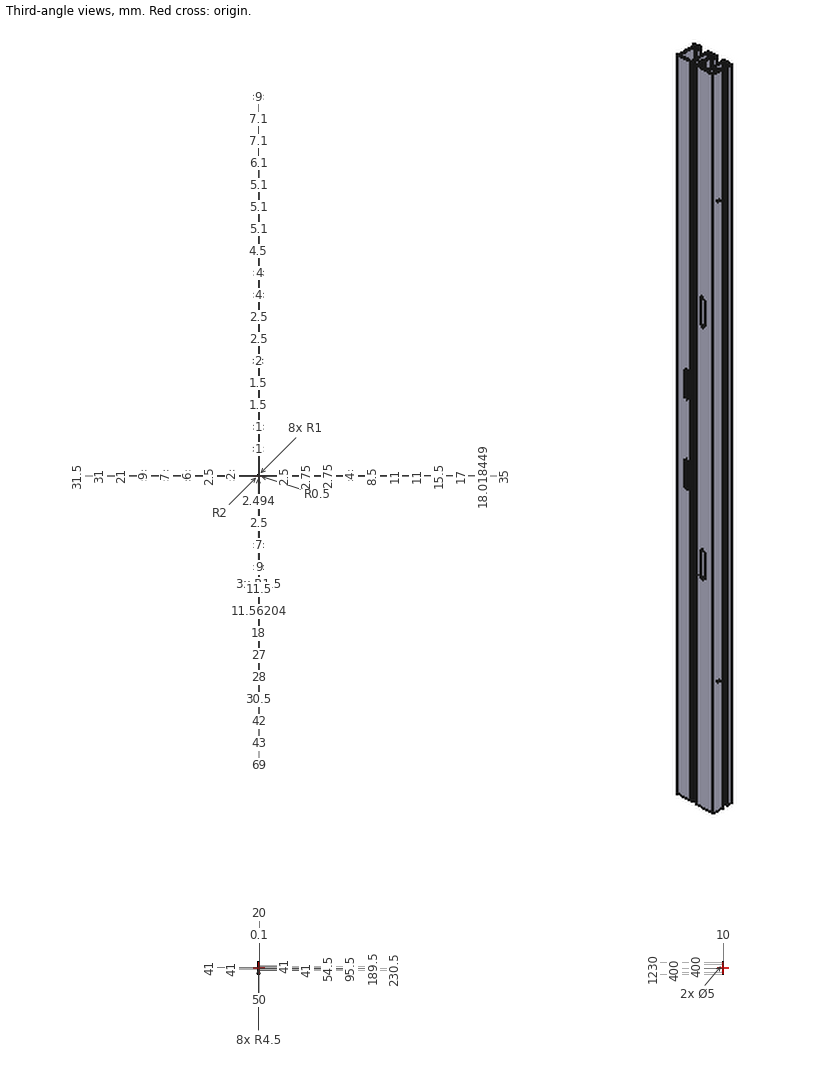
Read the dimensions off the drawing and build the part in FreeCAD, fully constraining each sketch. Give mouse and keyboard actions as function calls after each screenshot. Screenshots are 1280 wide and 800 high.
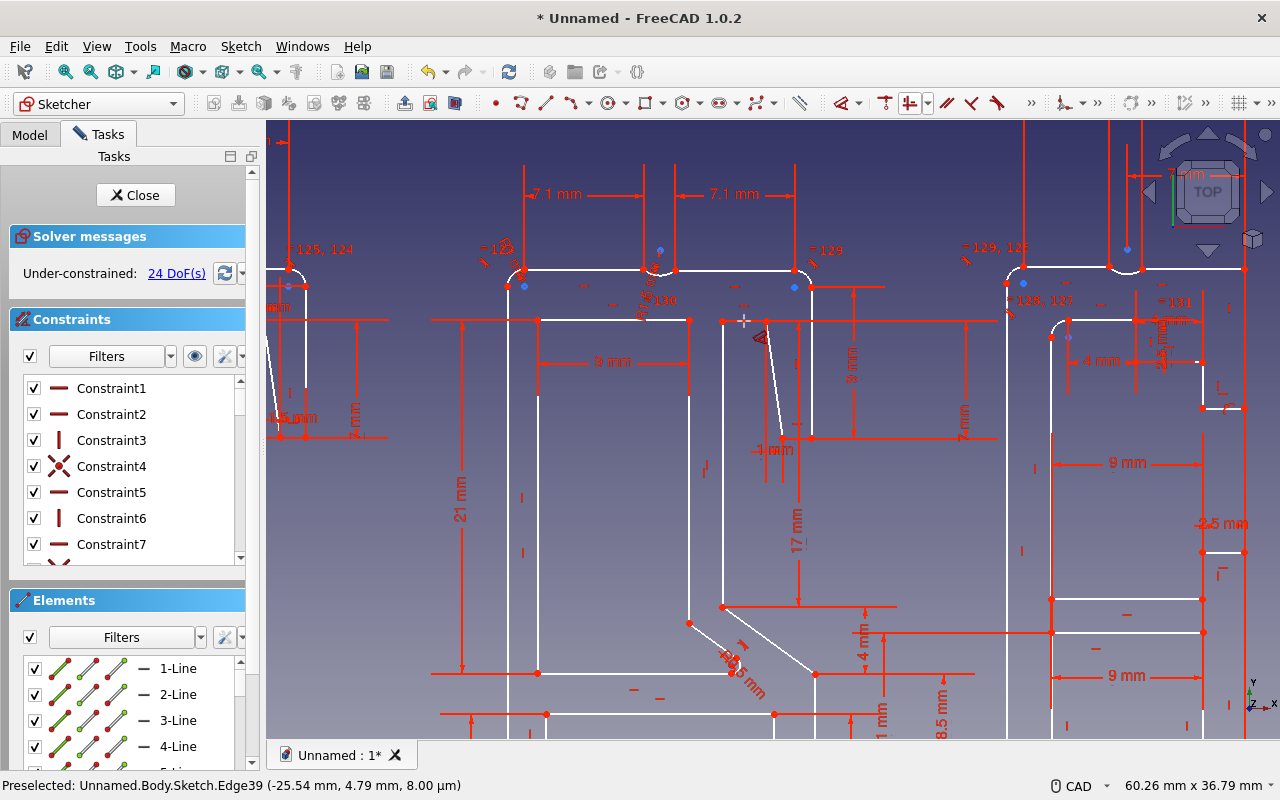
click(744, 321)
click(744, 287)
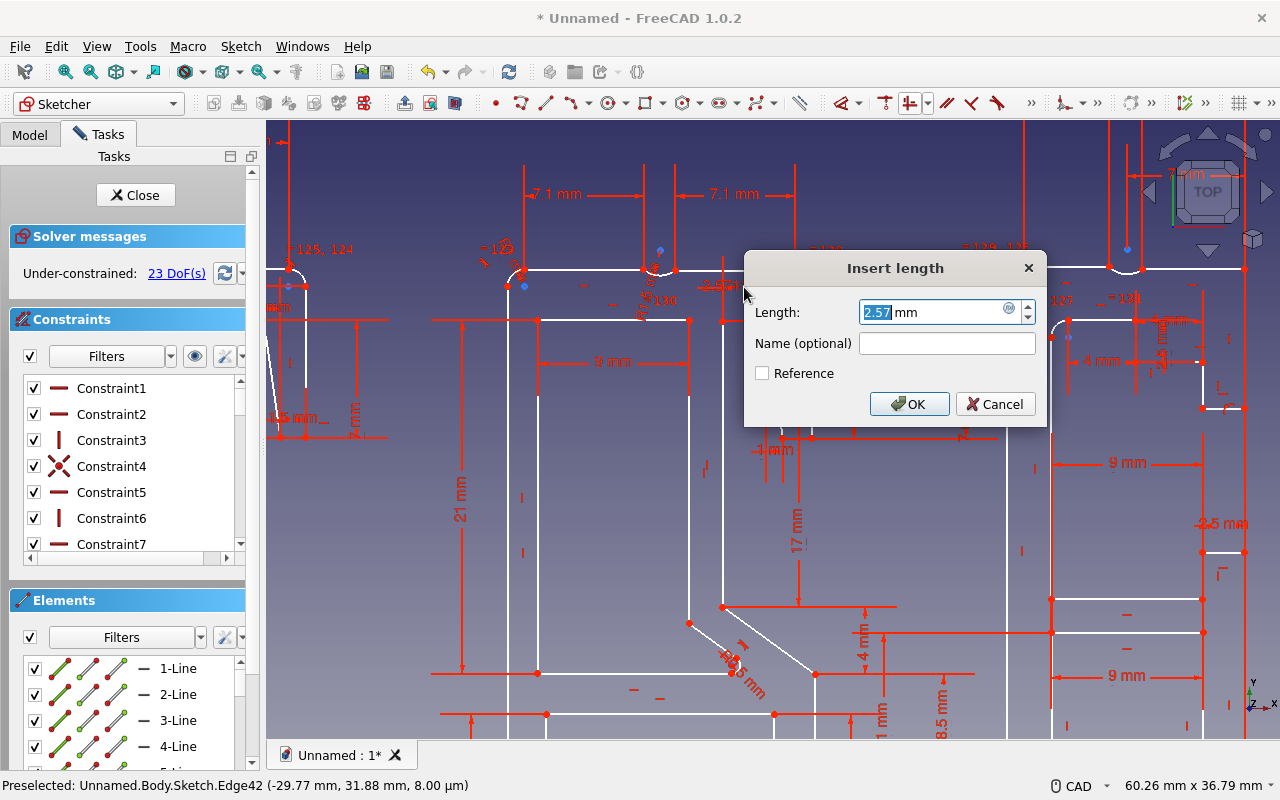
text(2.5)
key(Return)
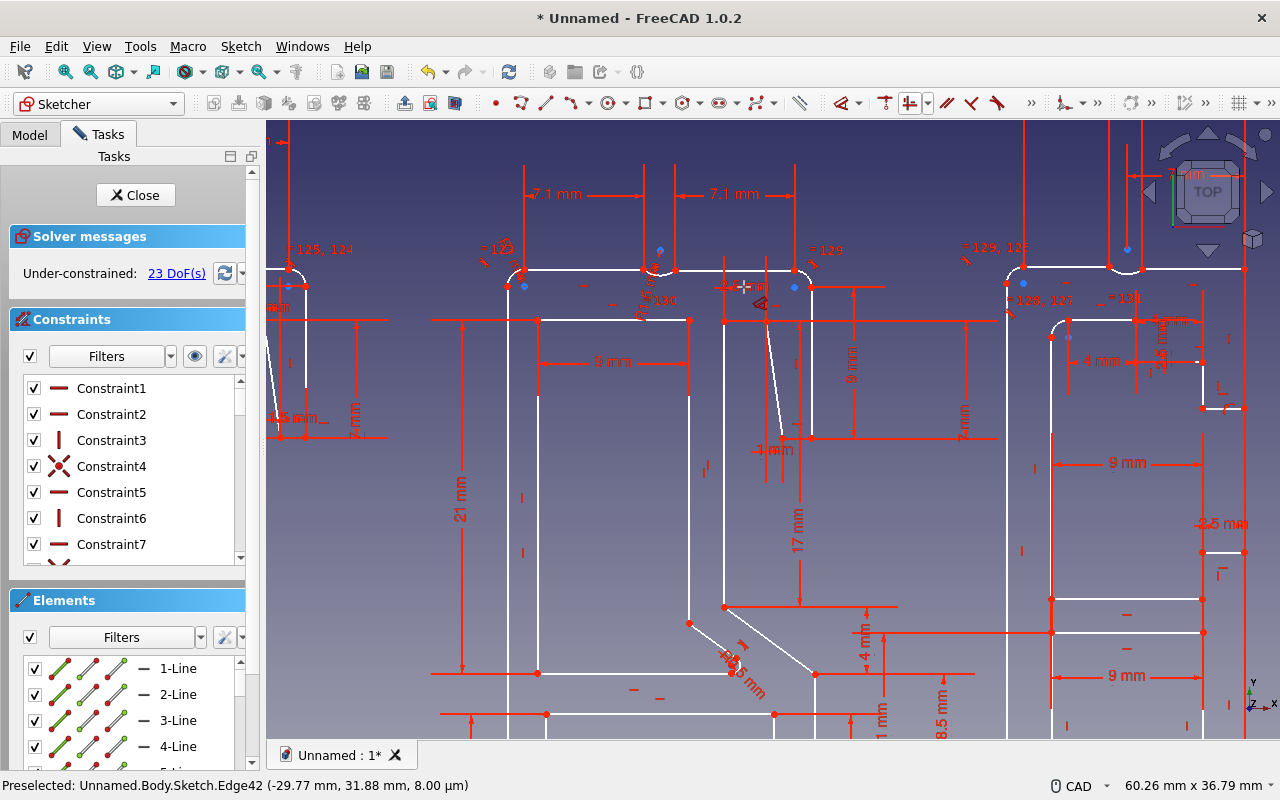
scroll(794, 439, up, 3)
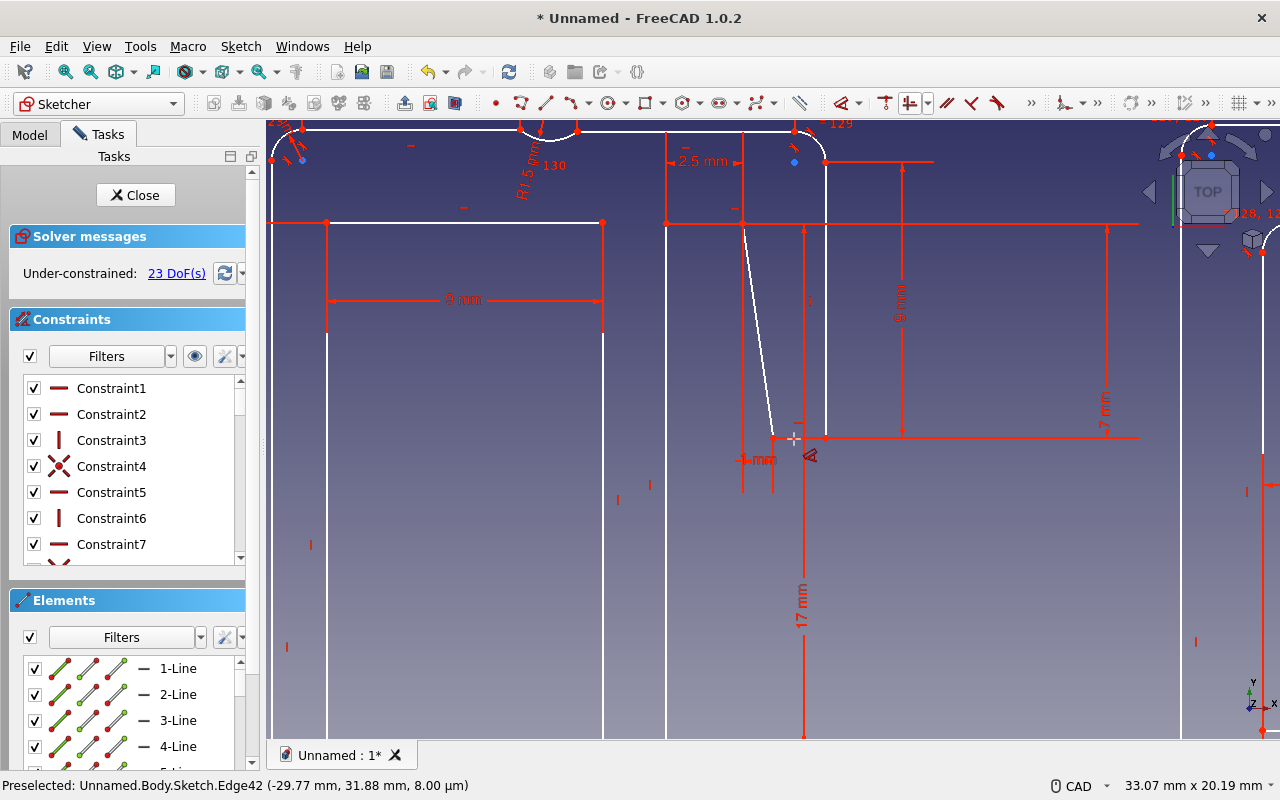
click(794, 438)
click(800, 404)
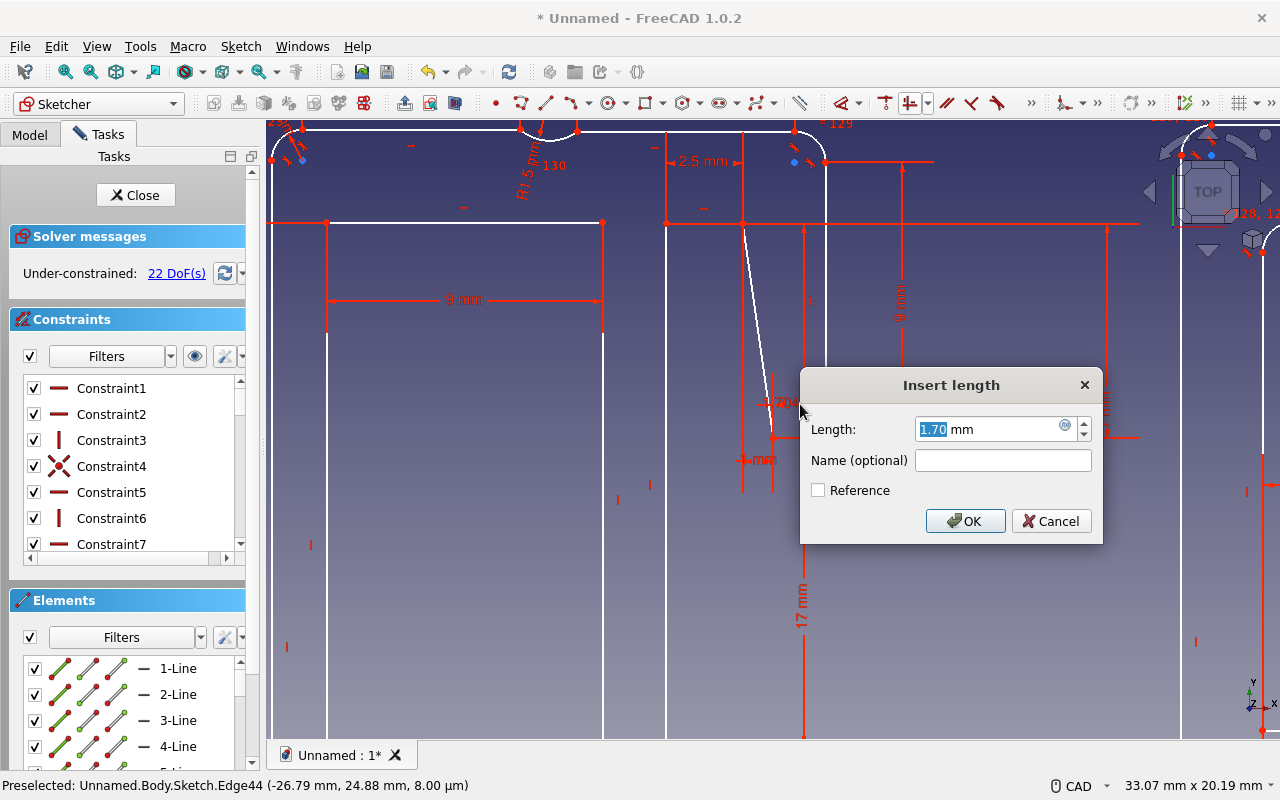
text(1.5)
key(Return)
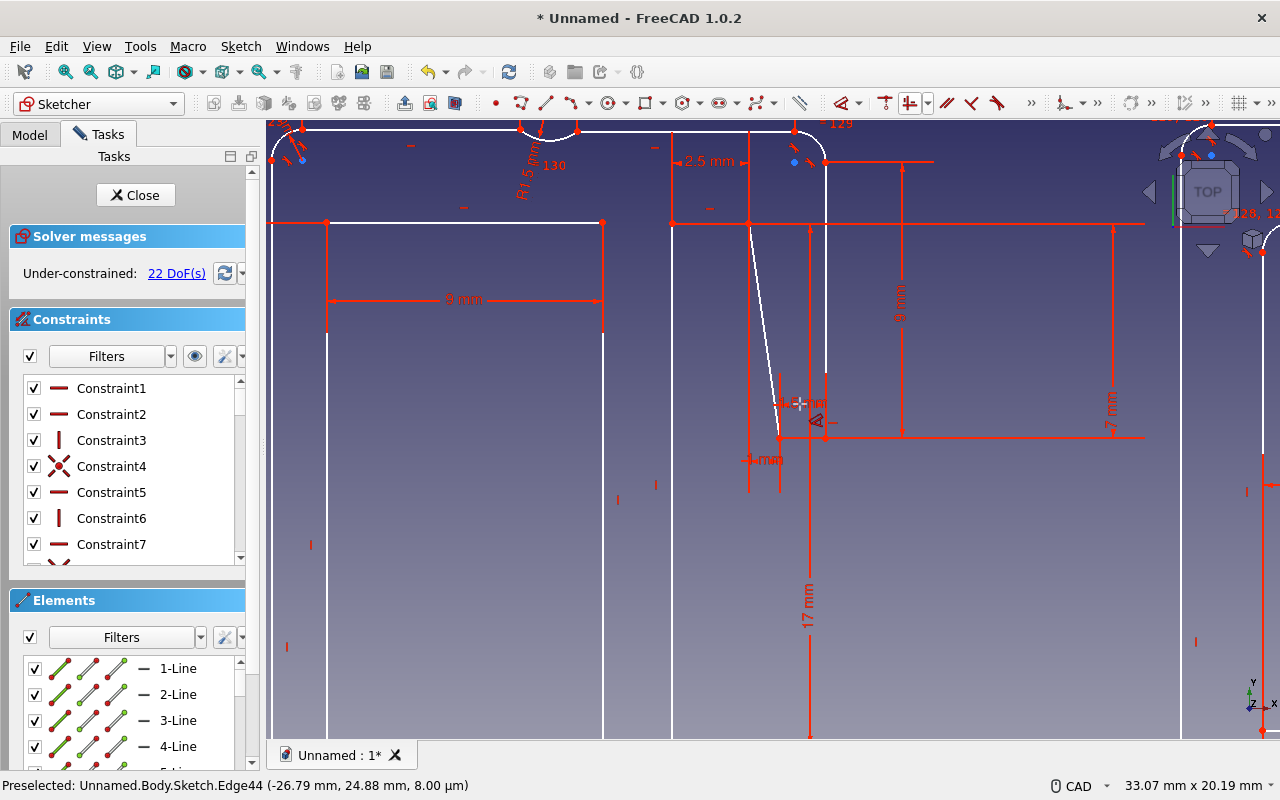
scroll(758, 353, down, 7)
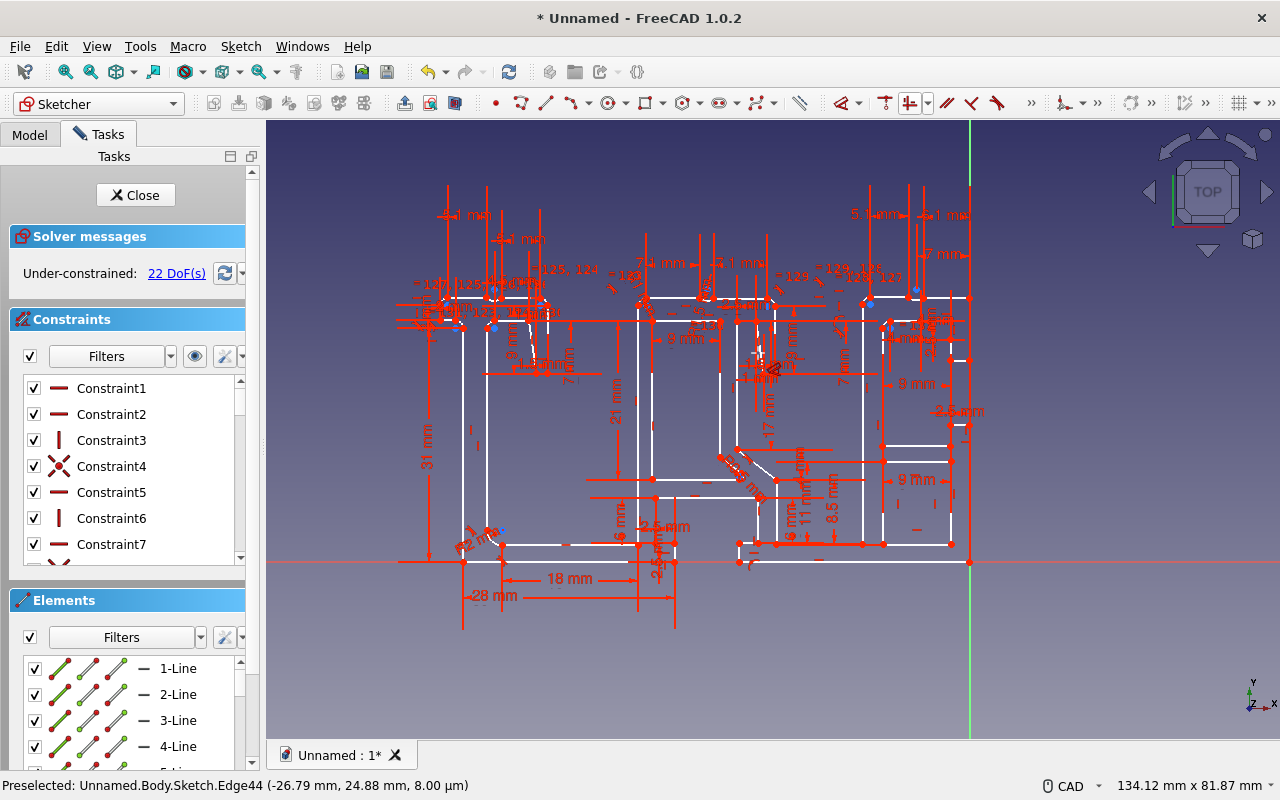
scroll(767, 299, up, 3)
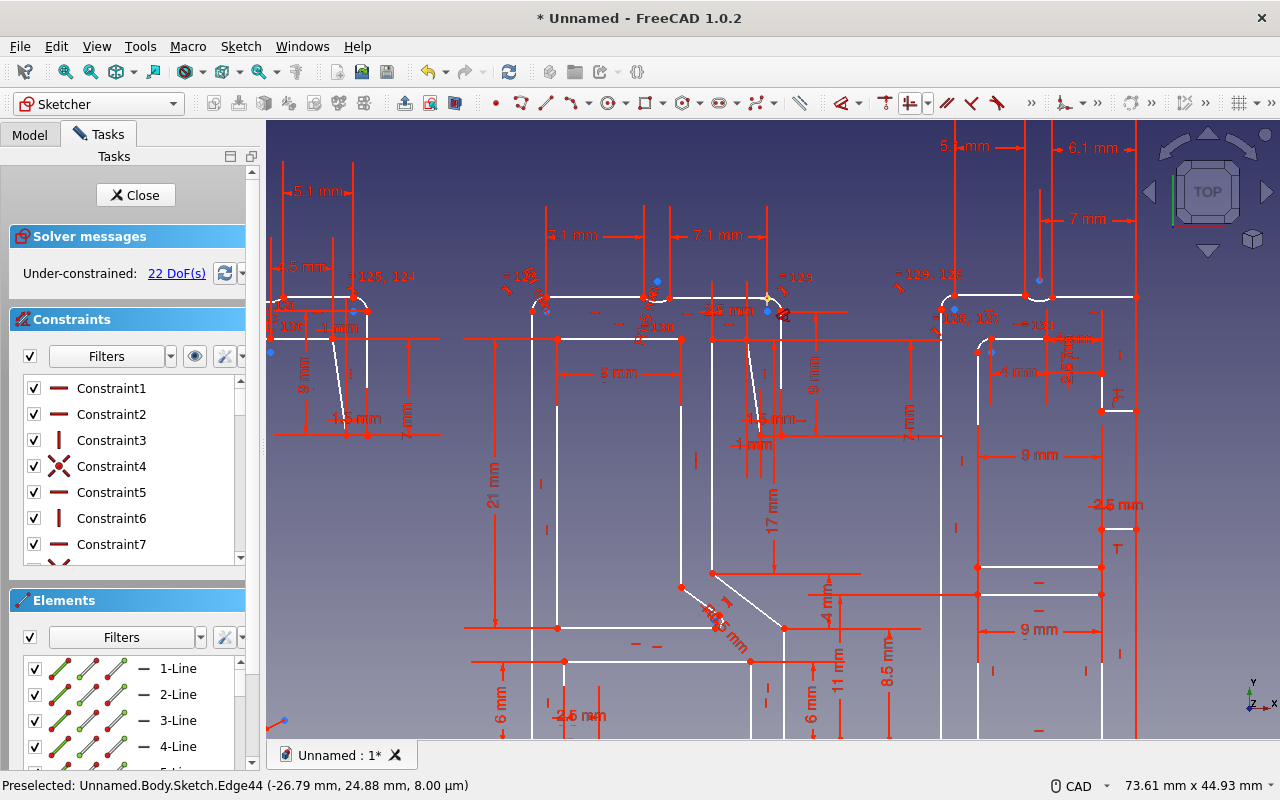
click(767, 298)
click(941, 264)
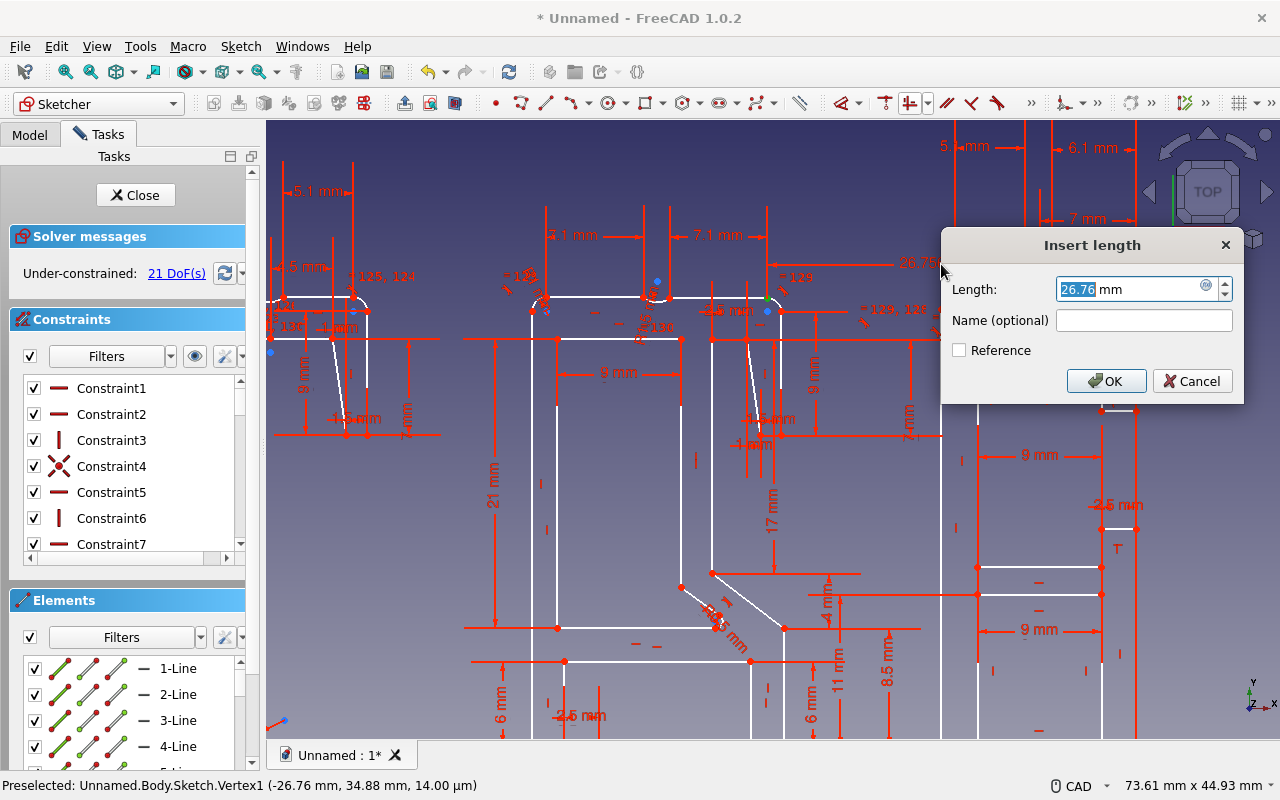
text(27)
key(Return)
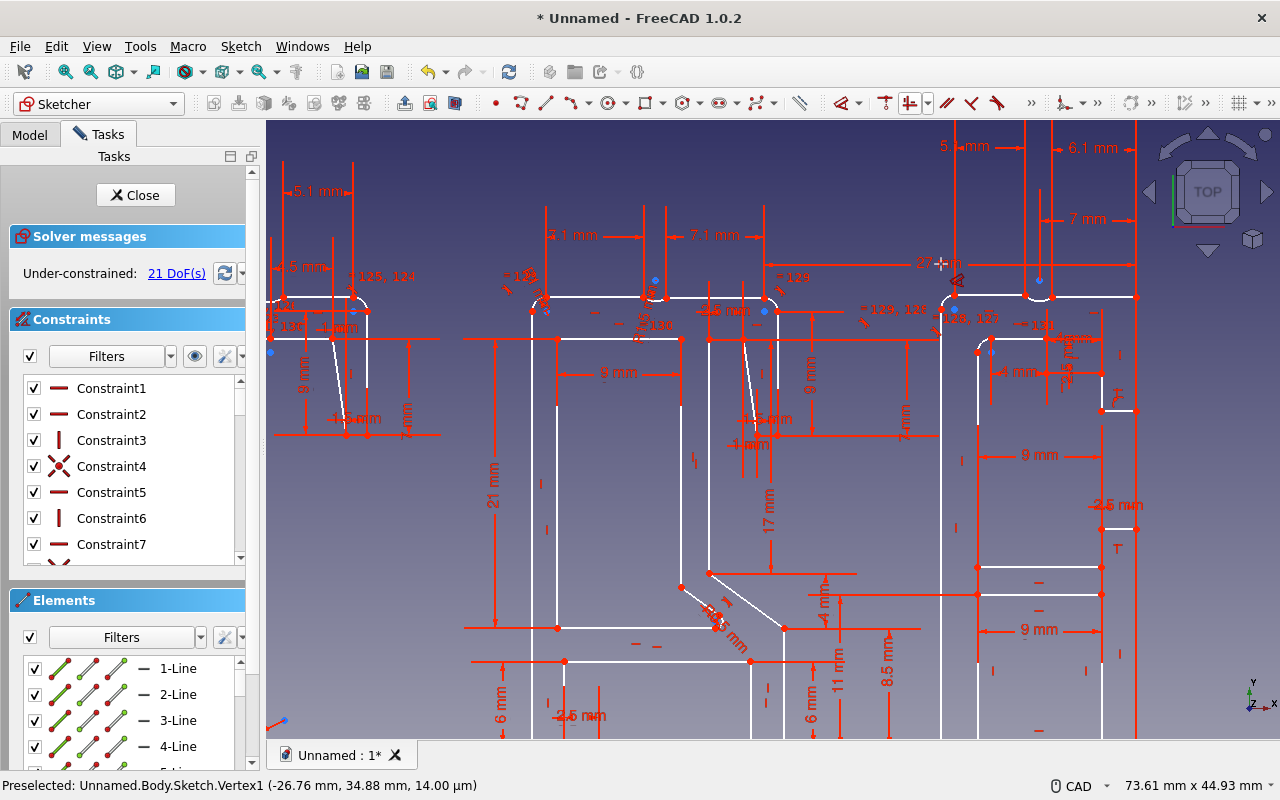
click(764, 298)
click(730, 360)